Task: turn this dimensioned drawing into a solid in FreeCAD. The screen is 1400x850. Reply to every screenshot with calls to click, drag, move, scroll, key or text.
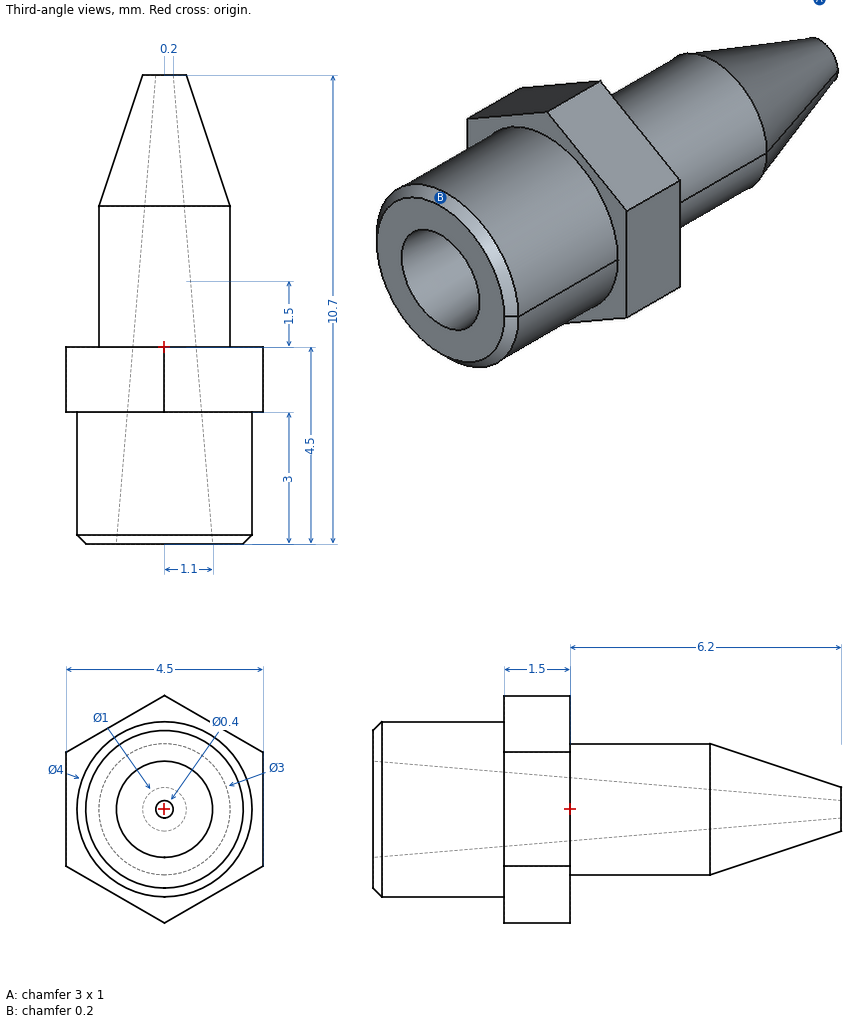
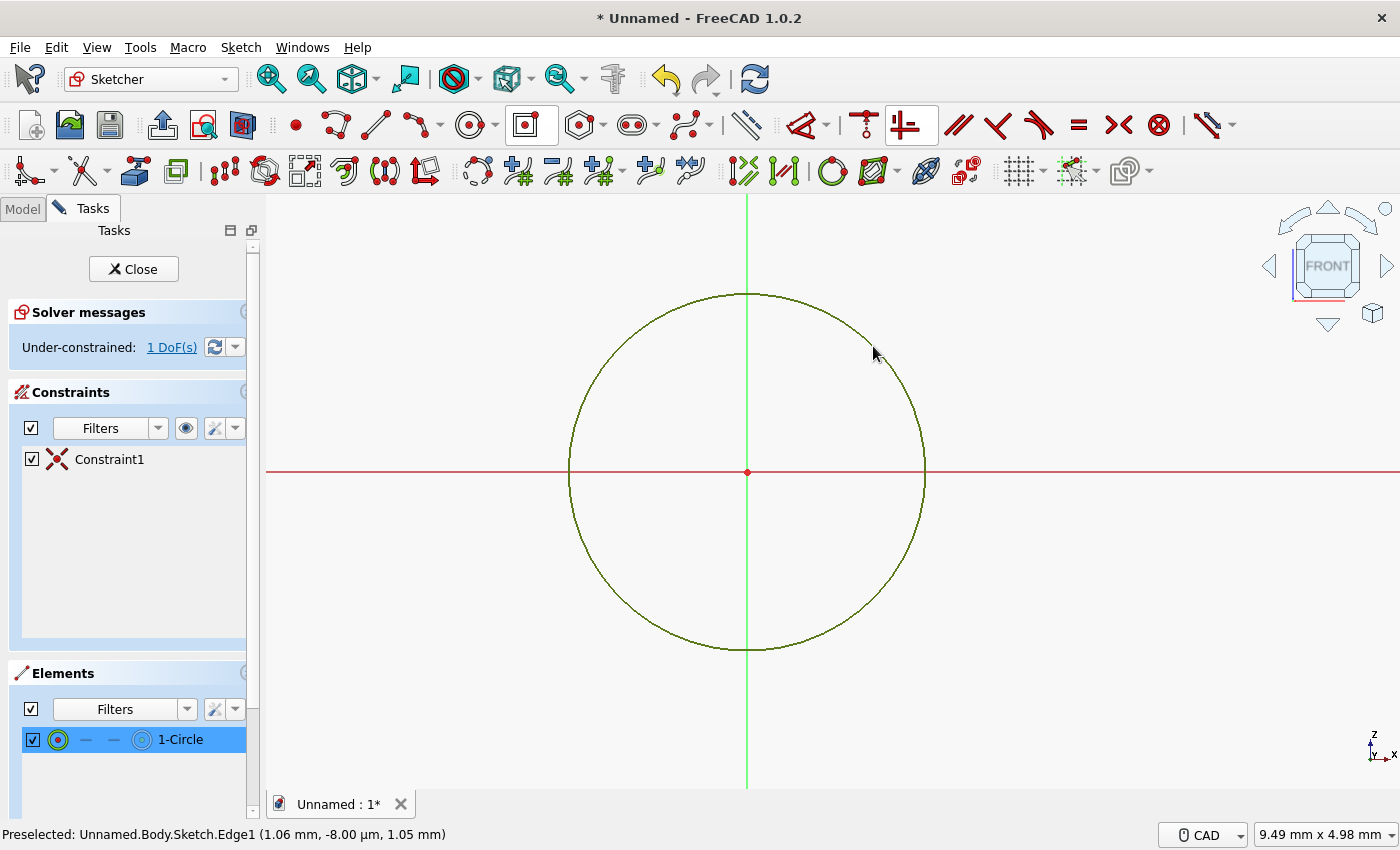
key(k)
key(o)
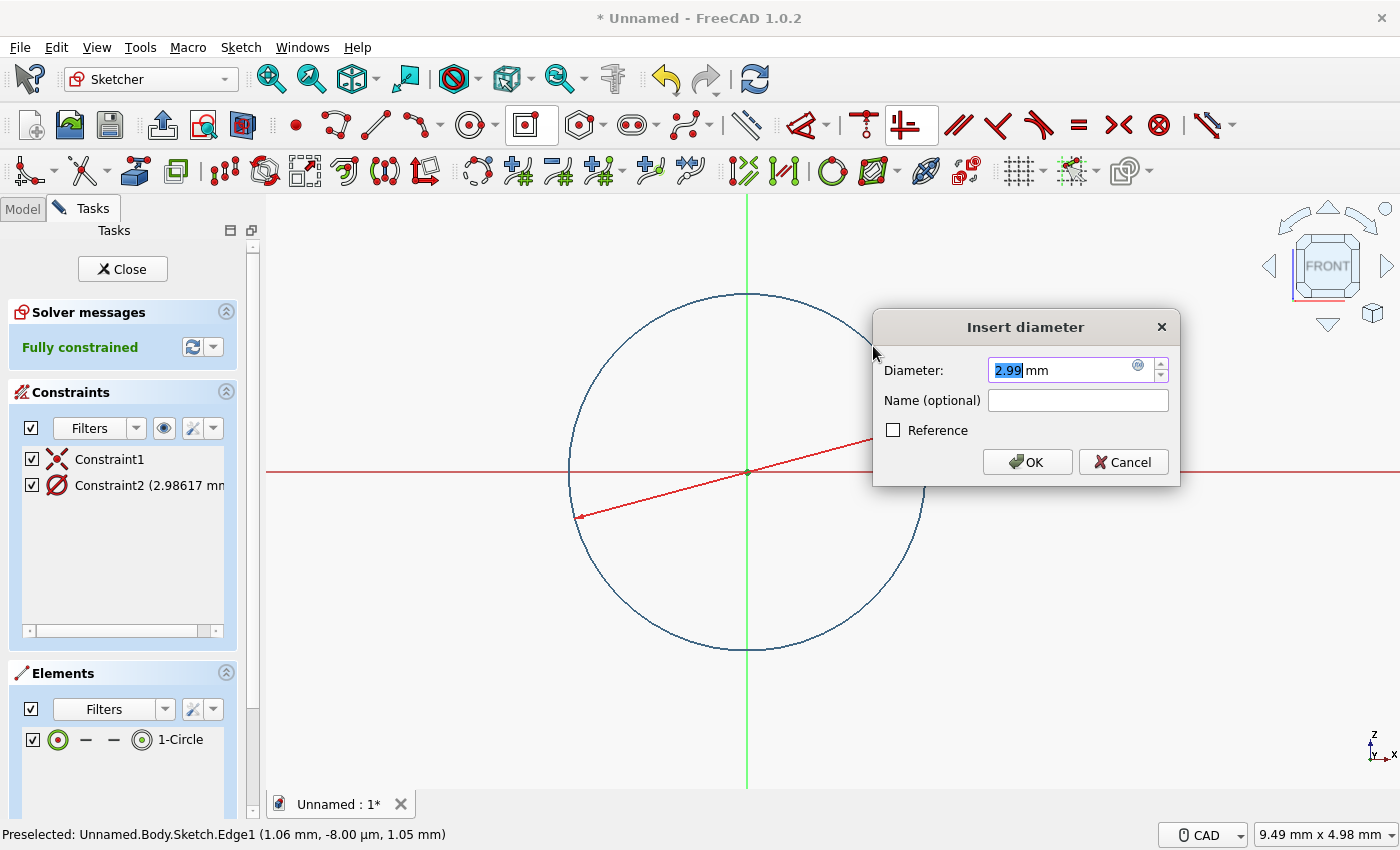
text(3)
key(Return)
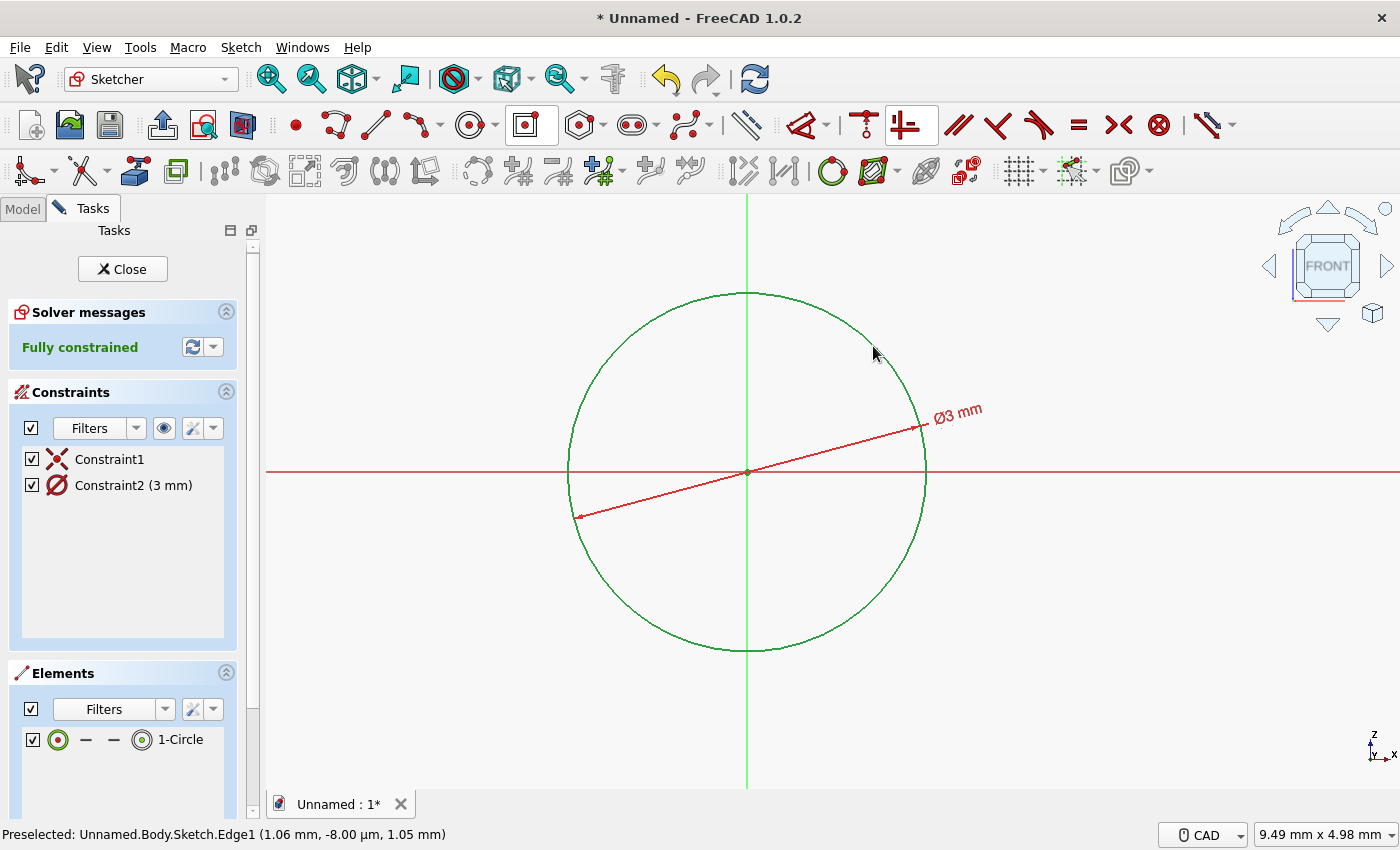
click(123, 269)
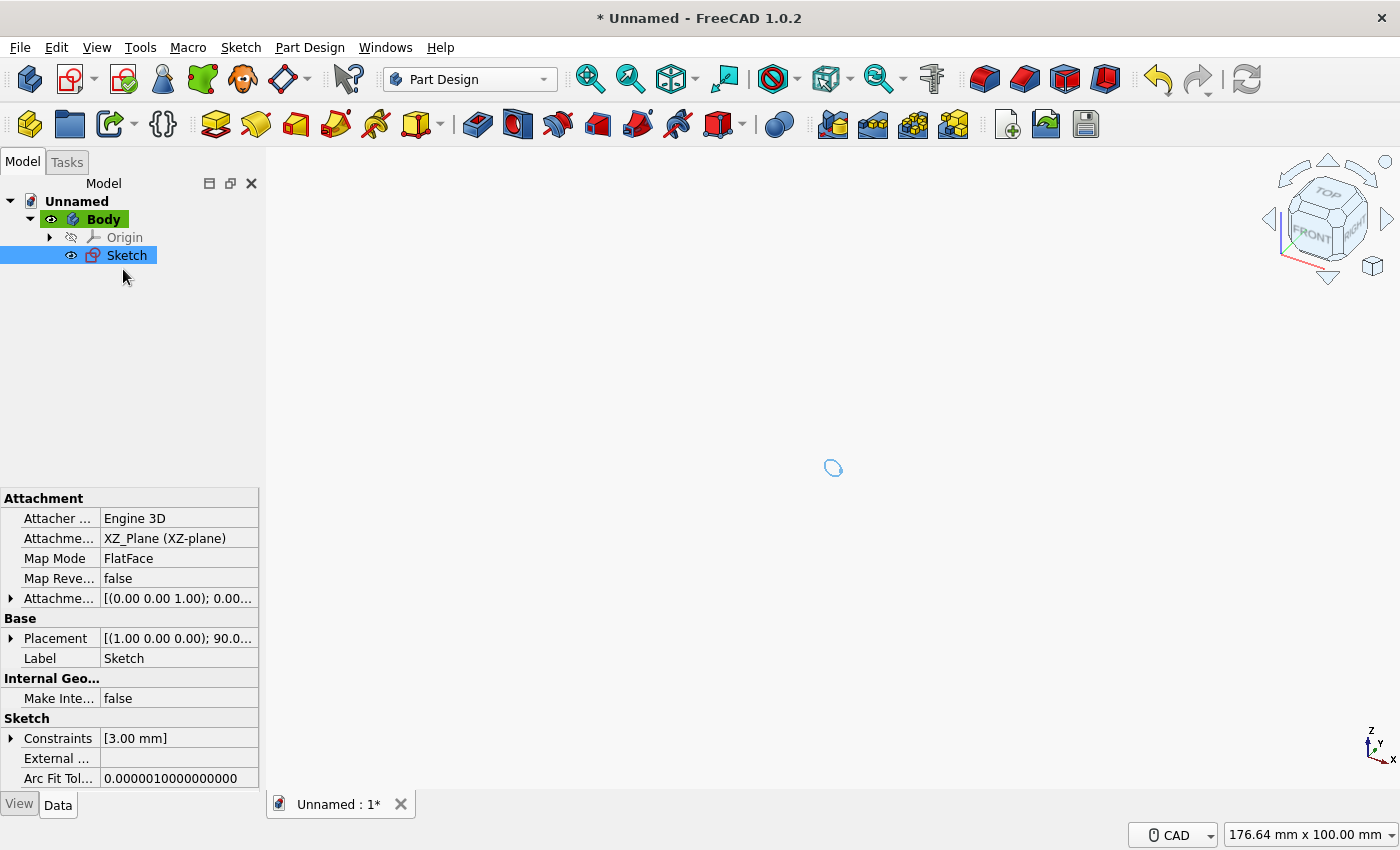
click(216, 124)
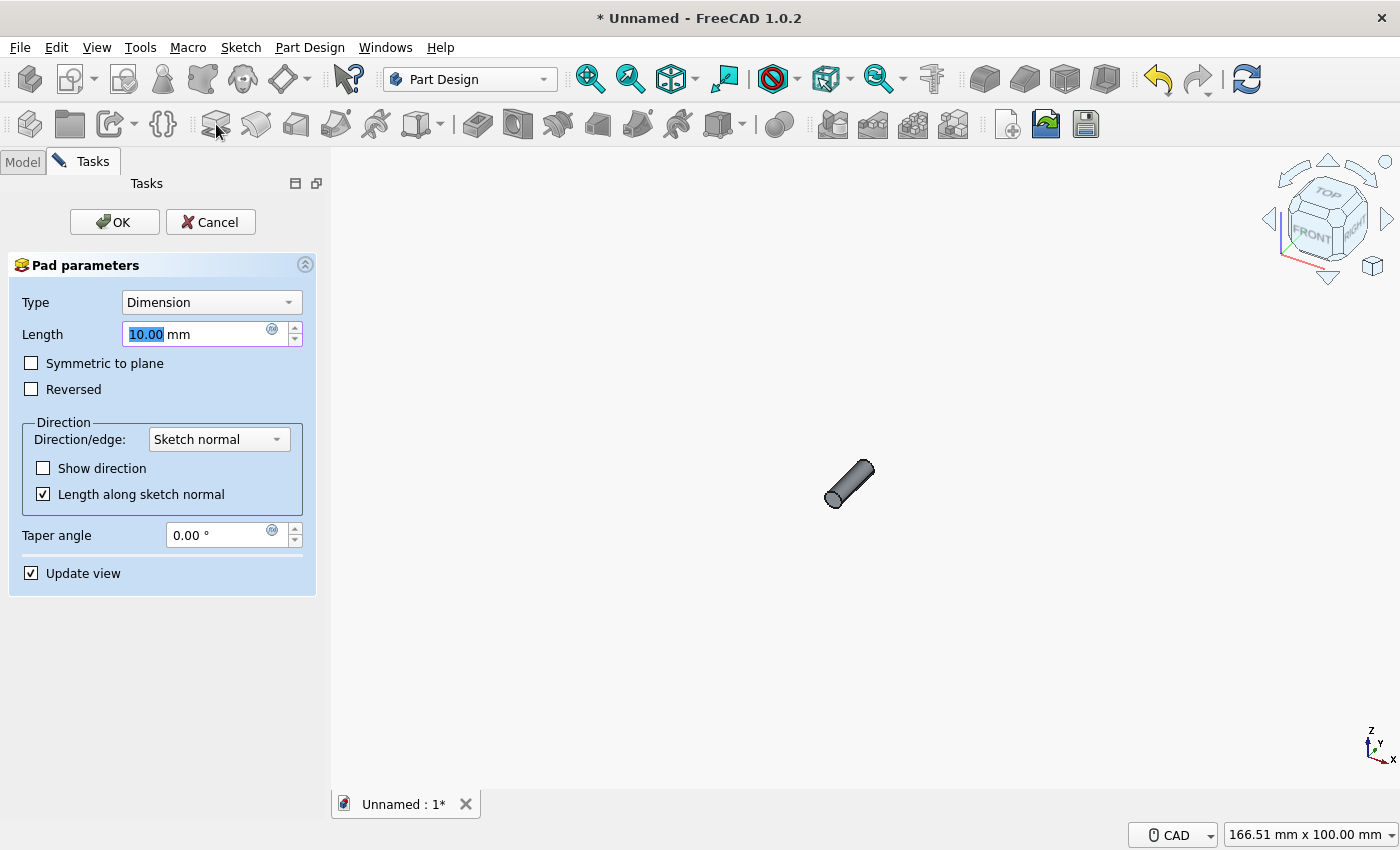
text(6.2)
key(Tab)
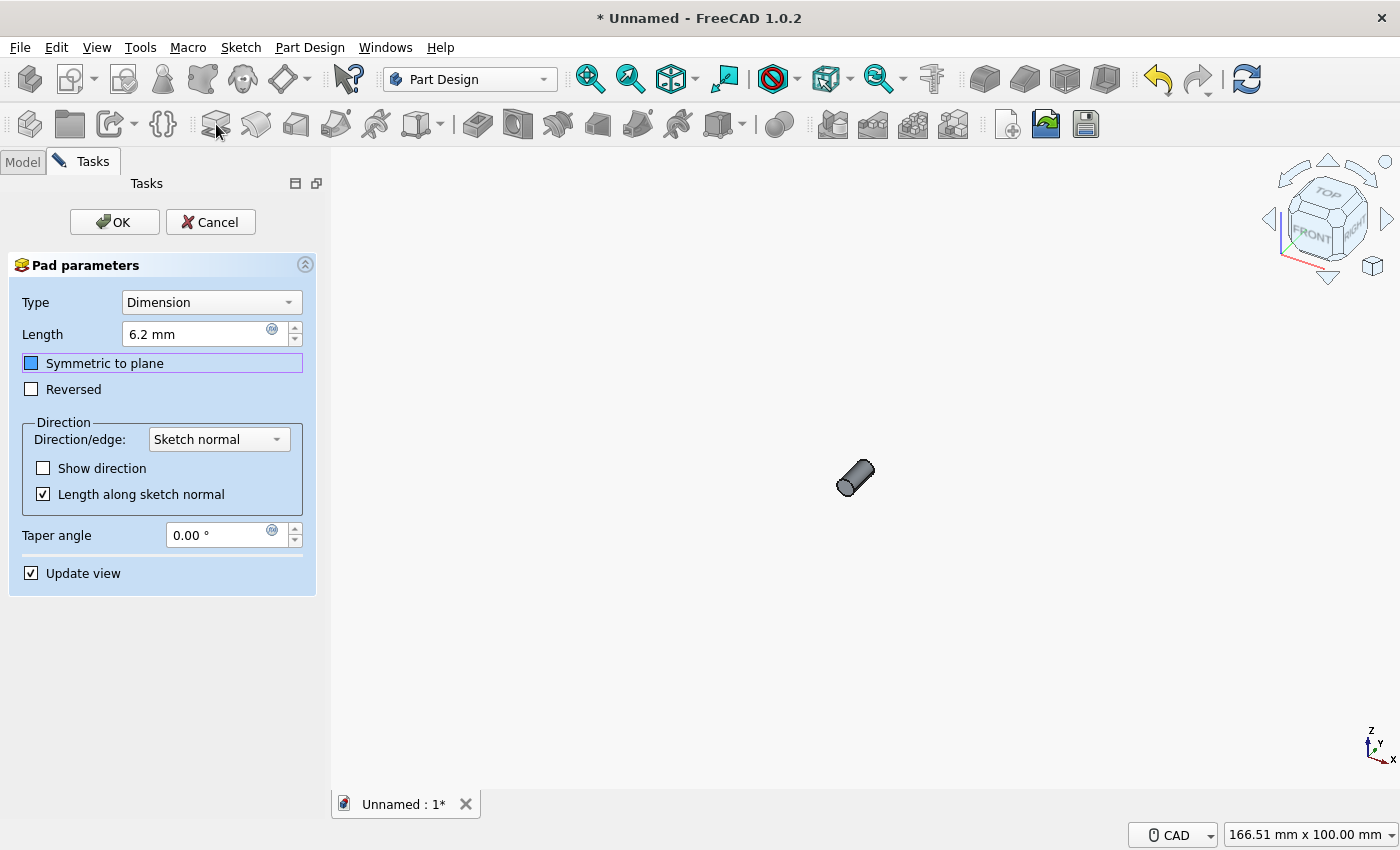
click(30, 389)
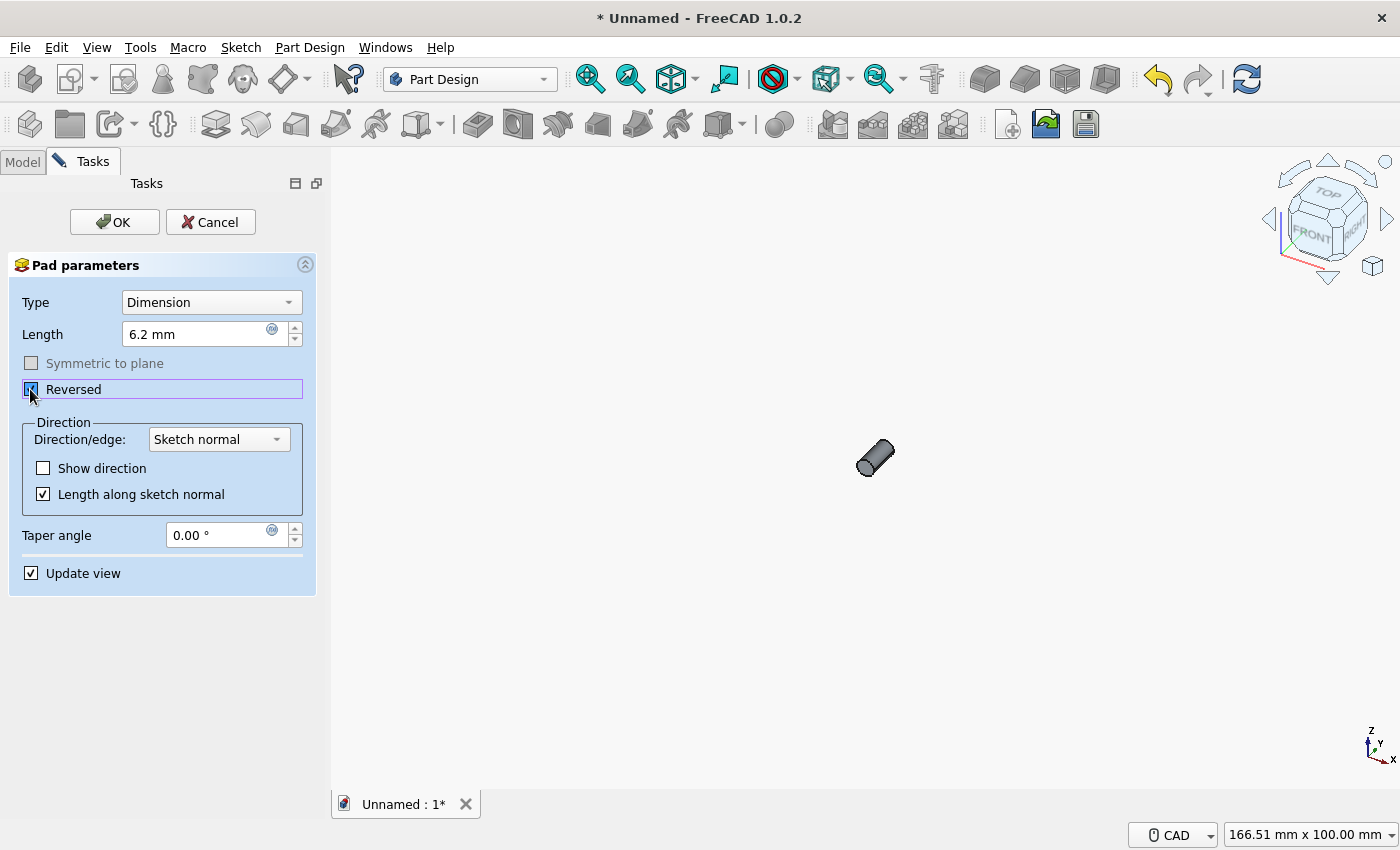
click(115, 222)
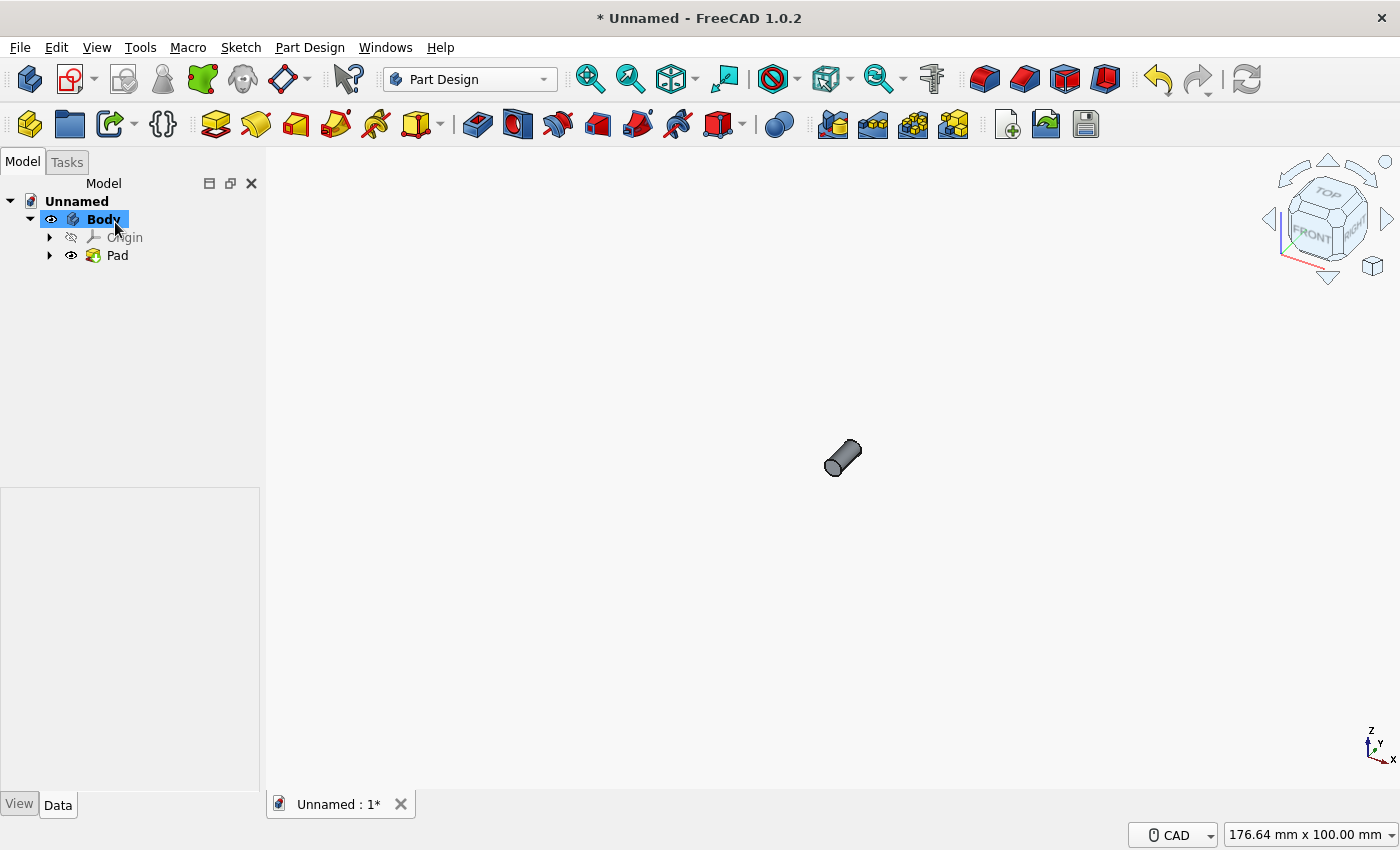
click(592, 80)